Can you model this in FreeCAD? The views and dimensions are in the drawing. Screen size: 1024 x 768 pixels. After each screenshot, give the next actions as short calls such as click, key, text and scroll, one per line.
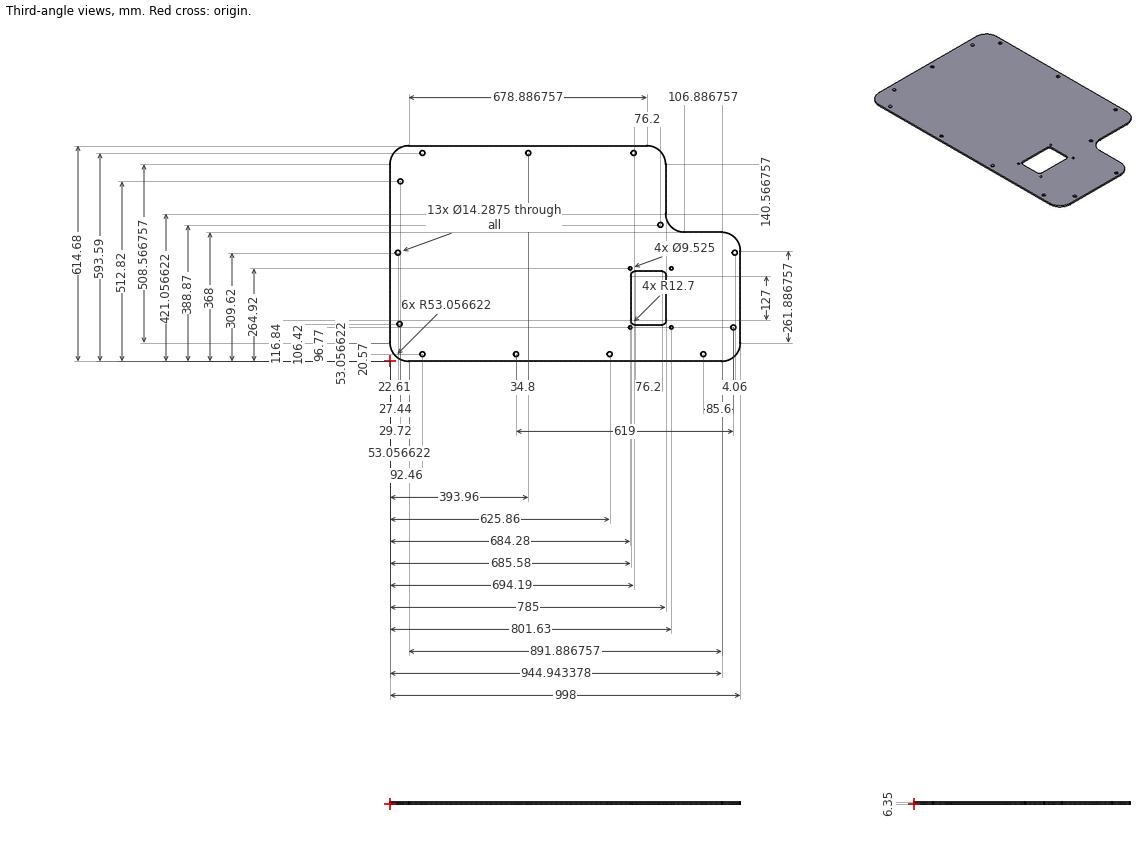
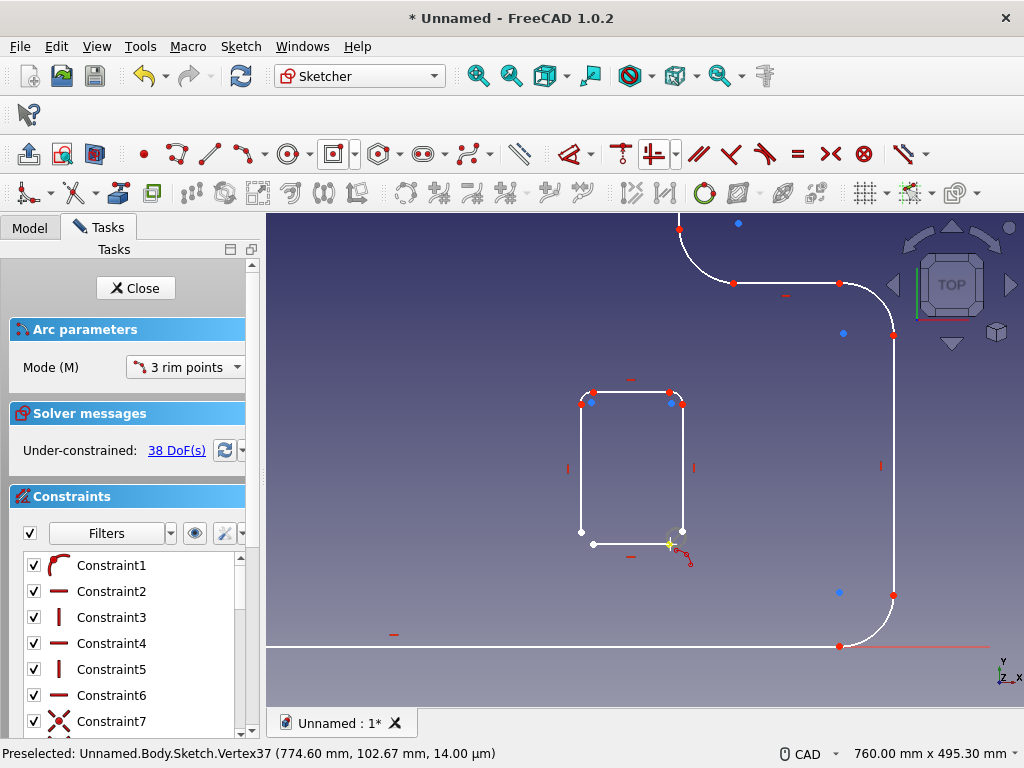
scroll(678, 539, up, 8)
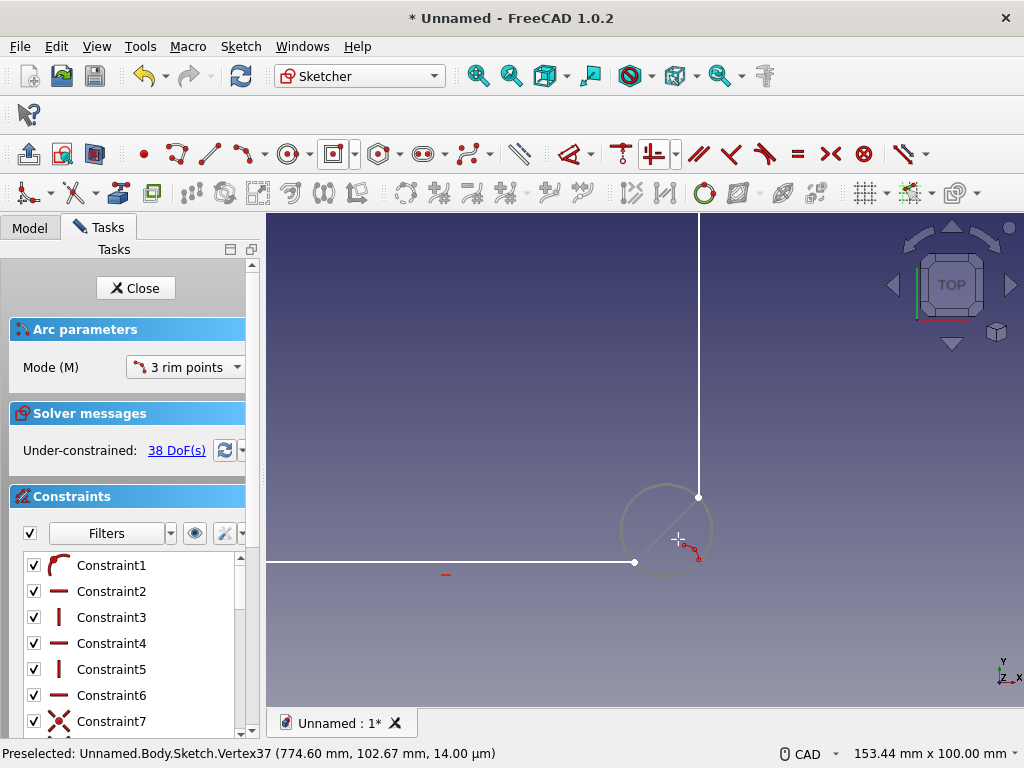
click(678, 537)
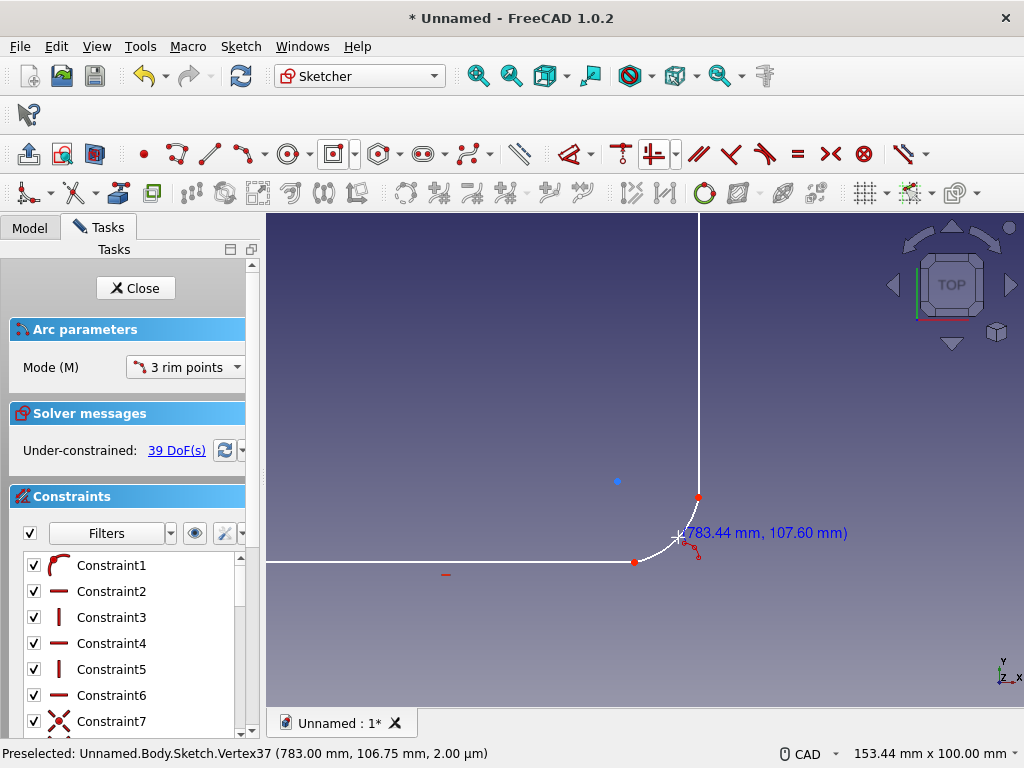
scroll(681, 533, down, 13)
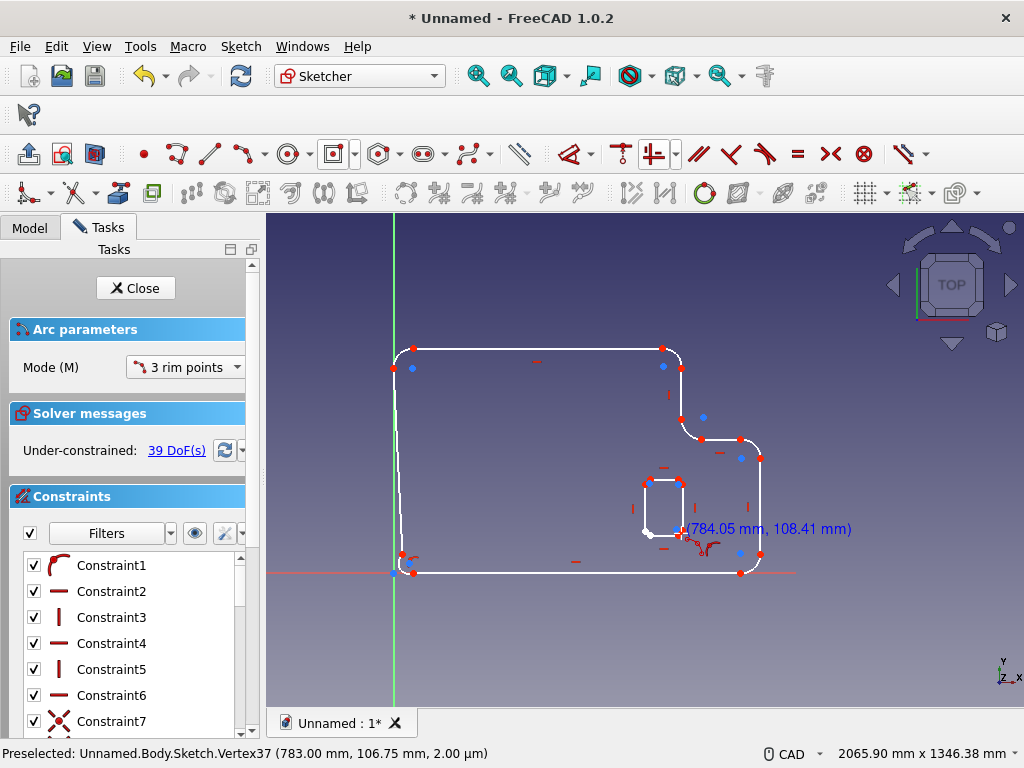
scroll(650, 535, up, 5)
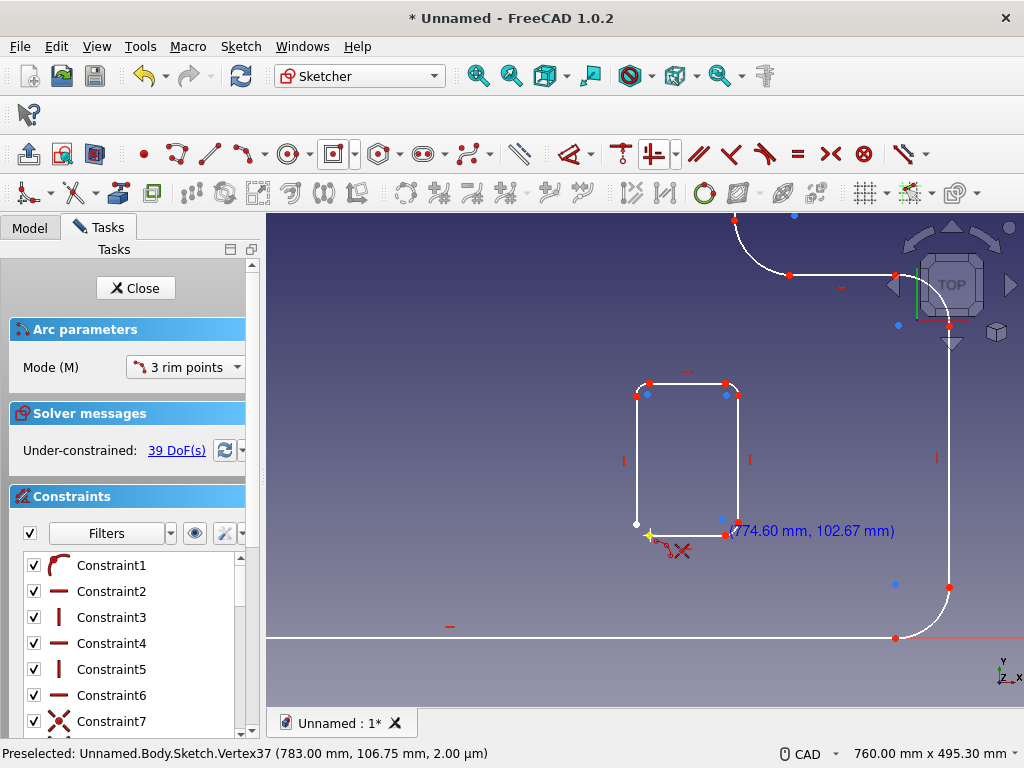
click(649, 536)
click(637, 524)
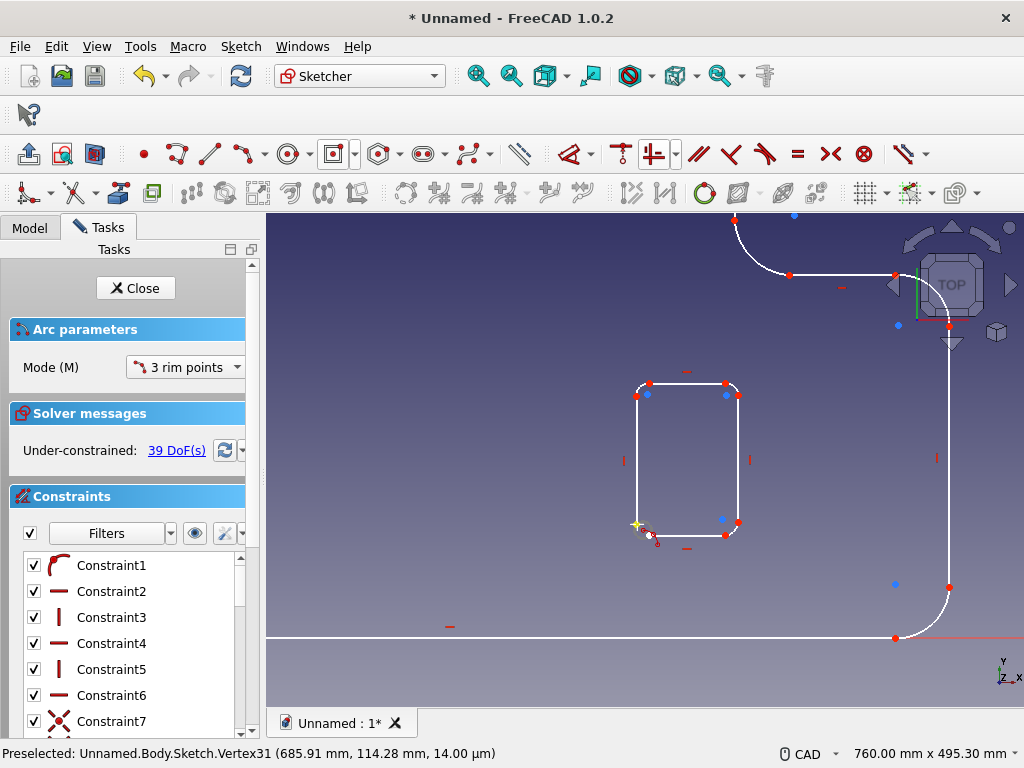
scroll(640, 531, up, 8)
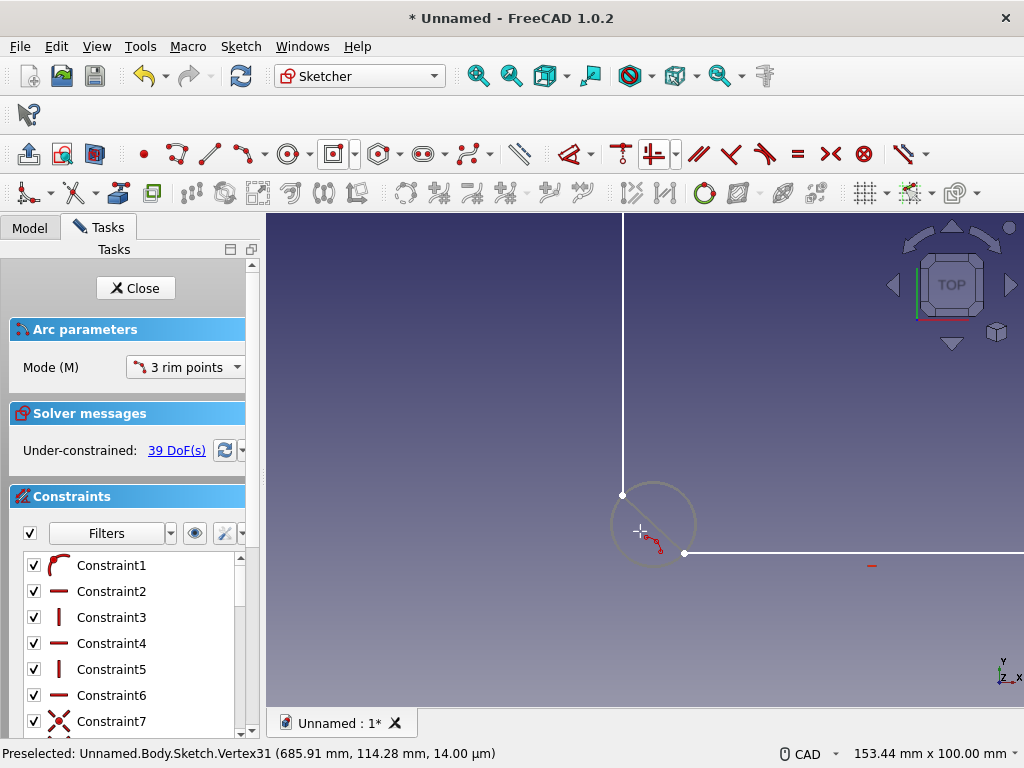
click(639, 528)
key(Escape)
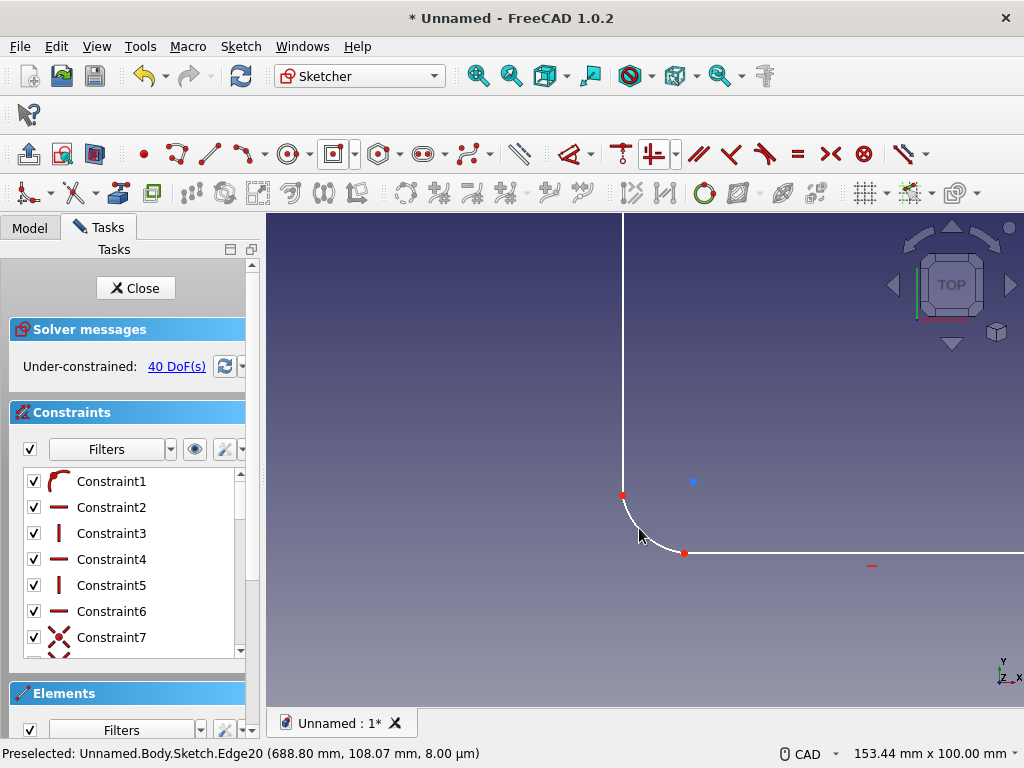
scroll(647, 534, down, 13)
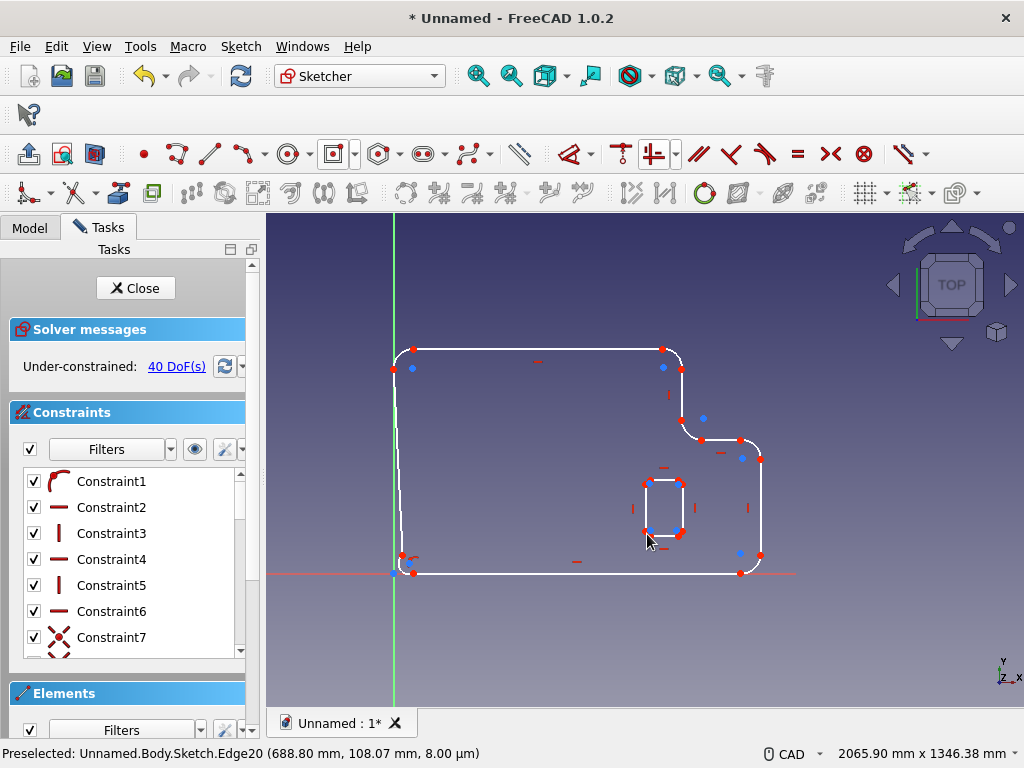
click(646, 518)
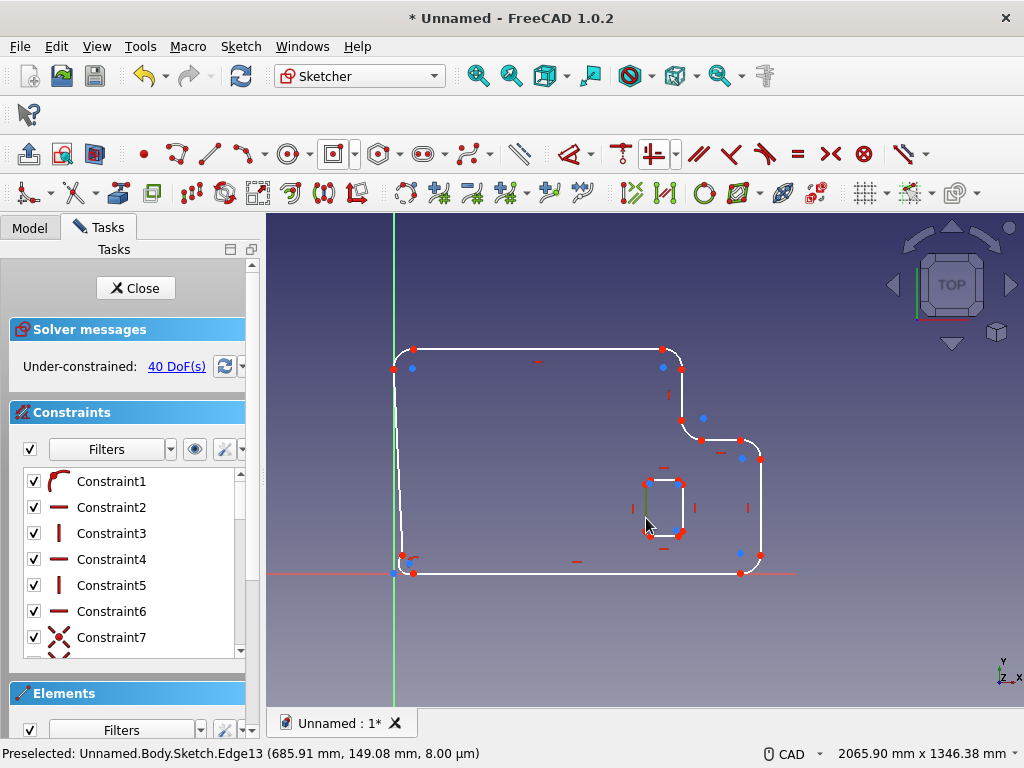
scroll(647, 481, up, 7)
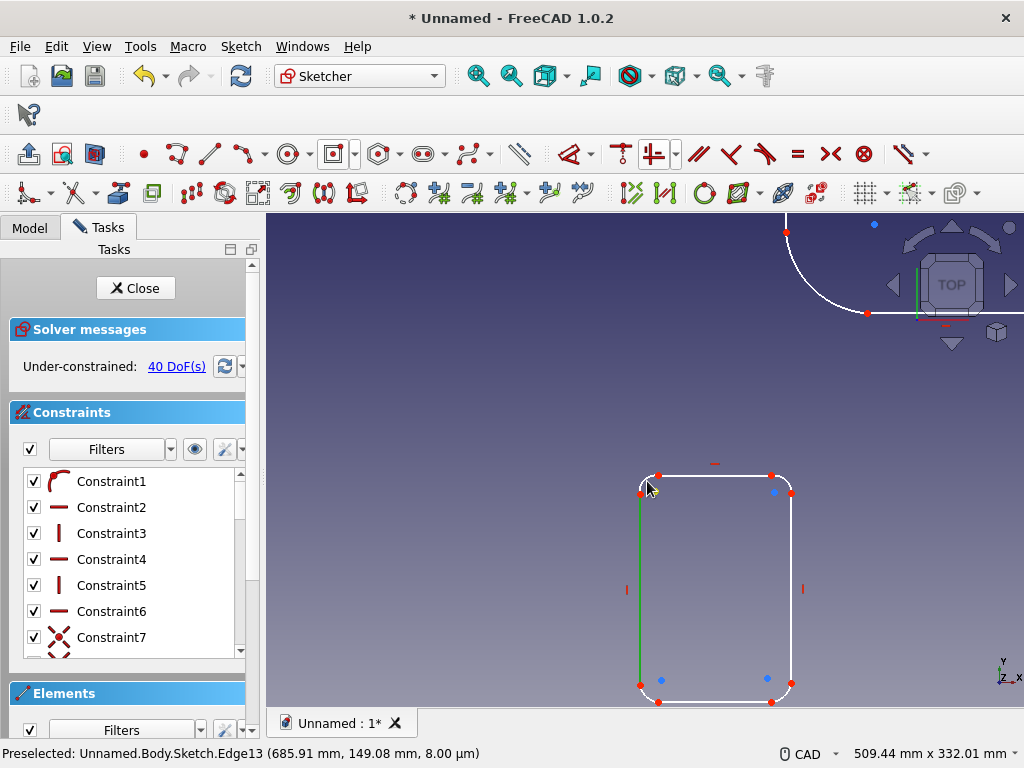
click(644, 480)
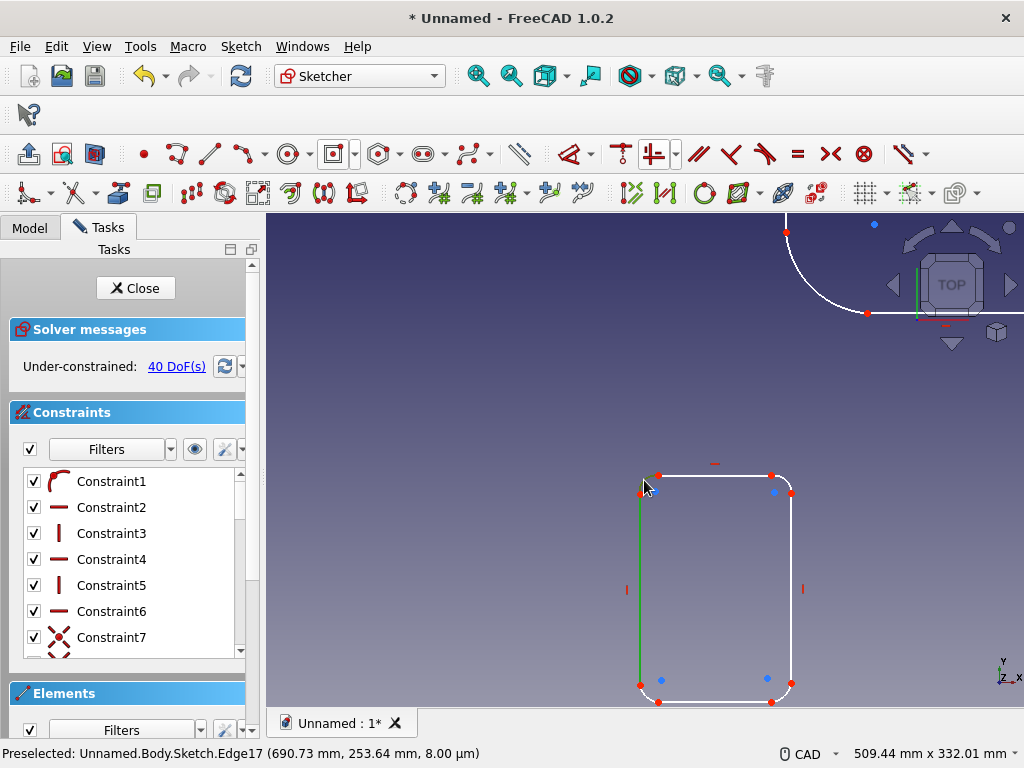
click(765, 154)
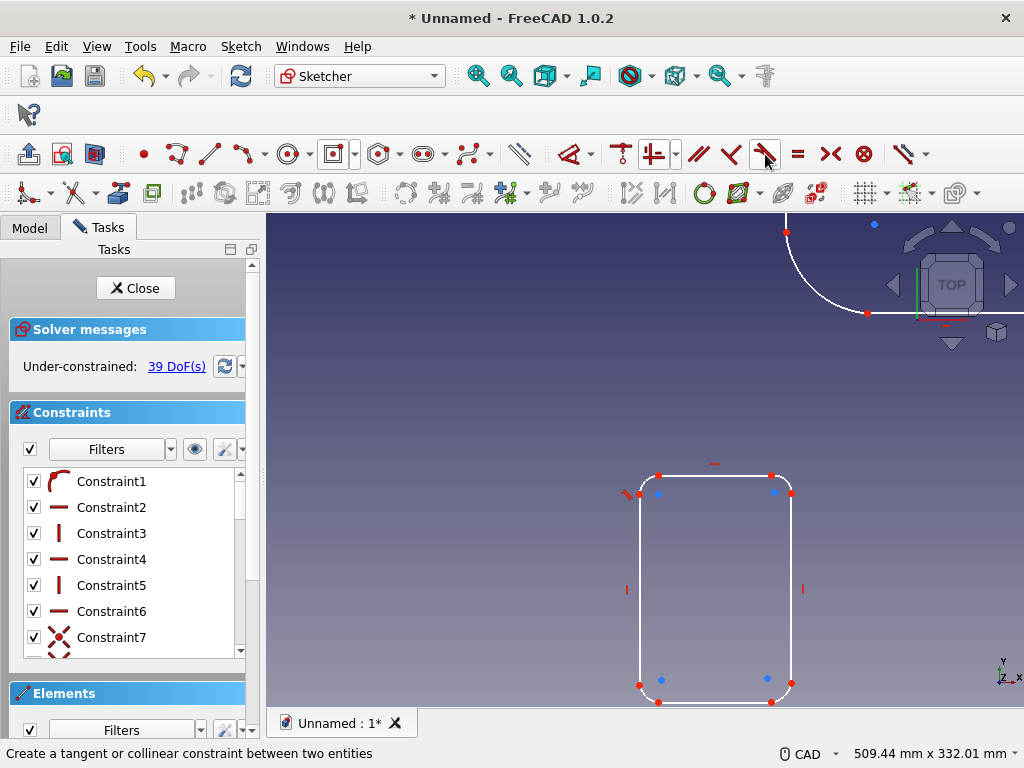
scroll(647, 480, down, 7)